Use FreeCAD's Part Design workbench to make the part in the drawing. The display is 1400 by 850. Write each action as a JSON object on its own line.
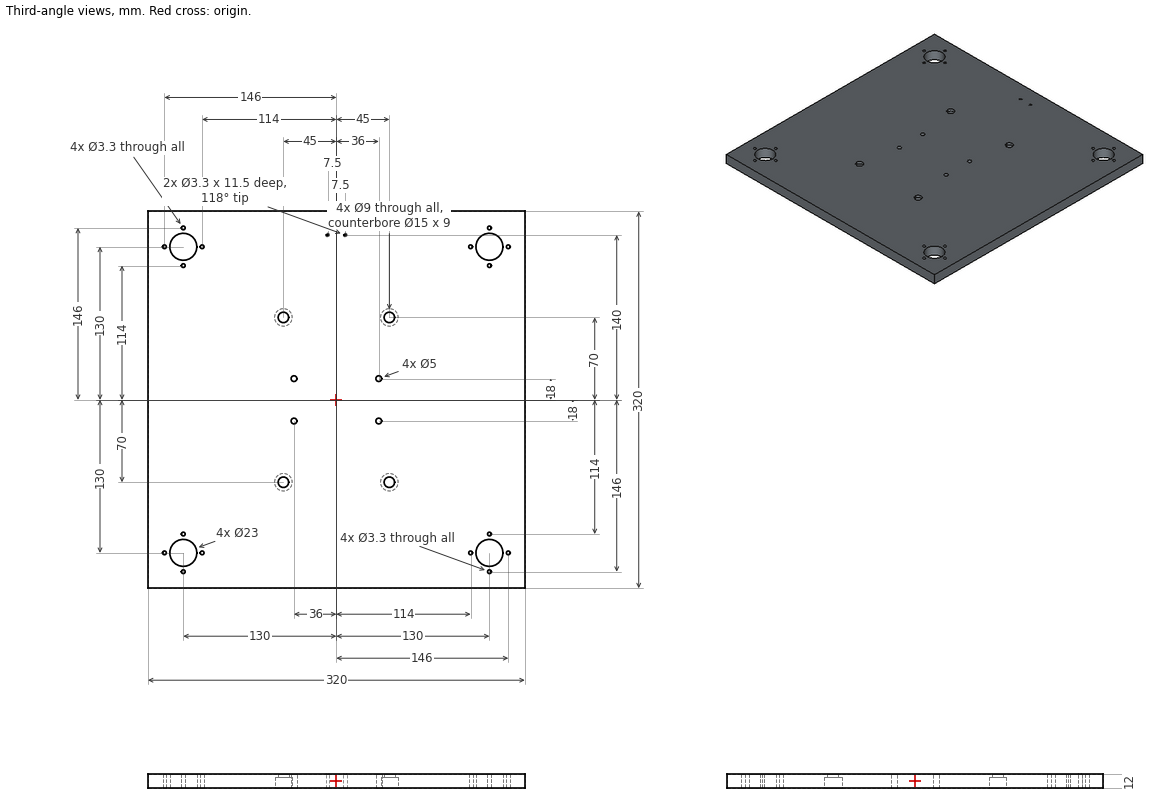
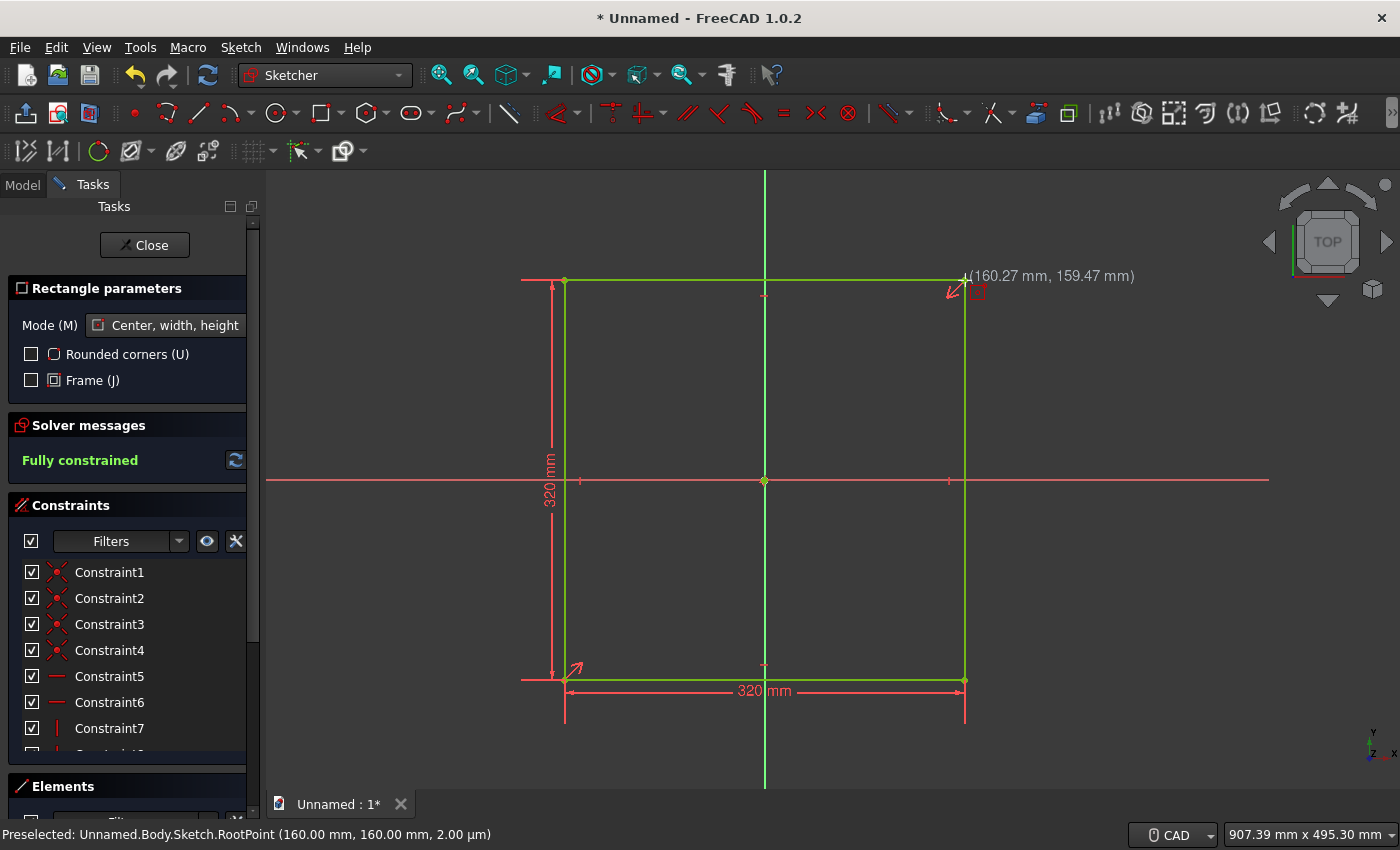
{"action": "left_click", "coordinate": [276, 114]}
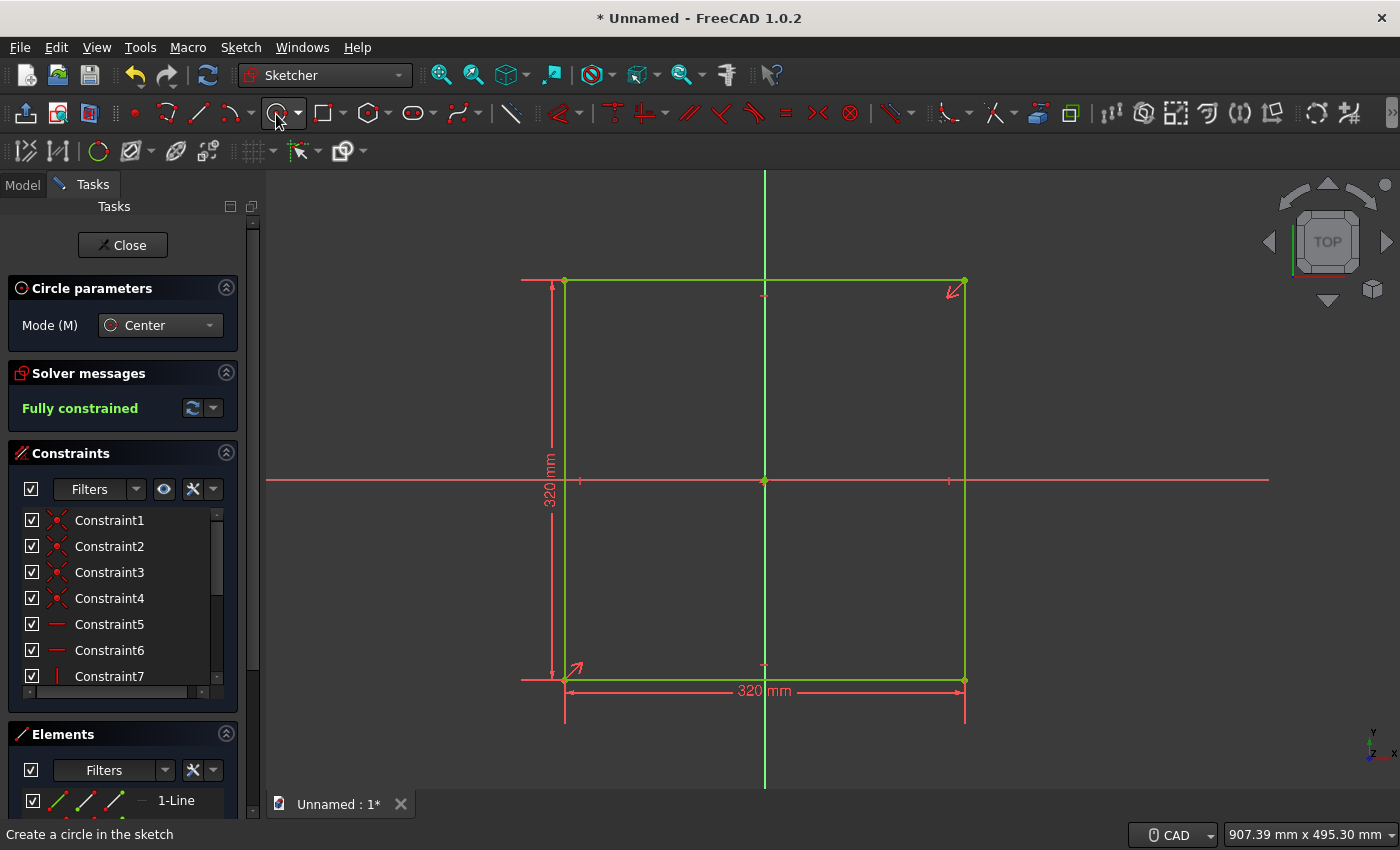
{"action": "scroll", "coordinate": [602, 643], "scroll_direction": "up", "scroll_amount": 3}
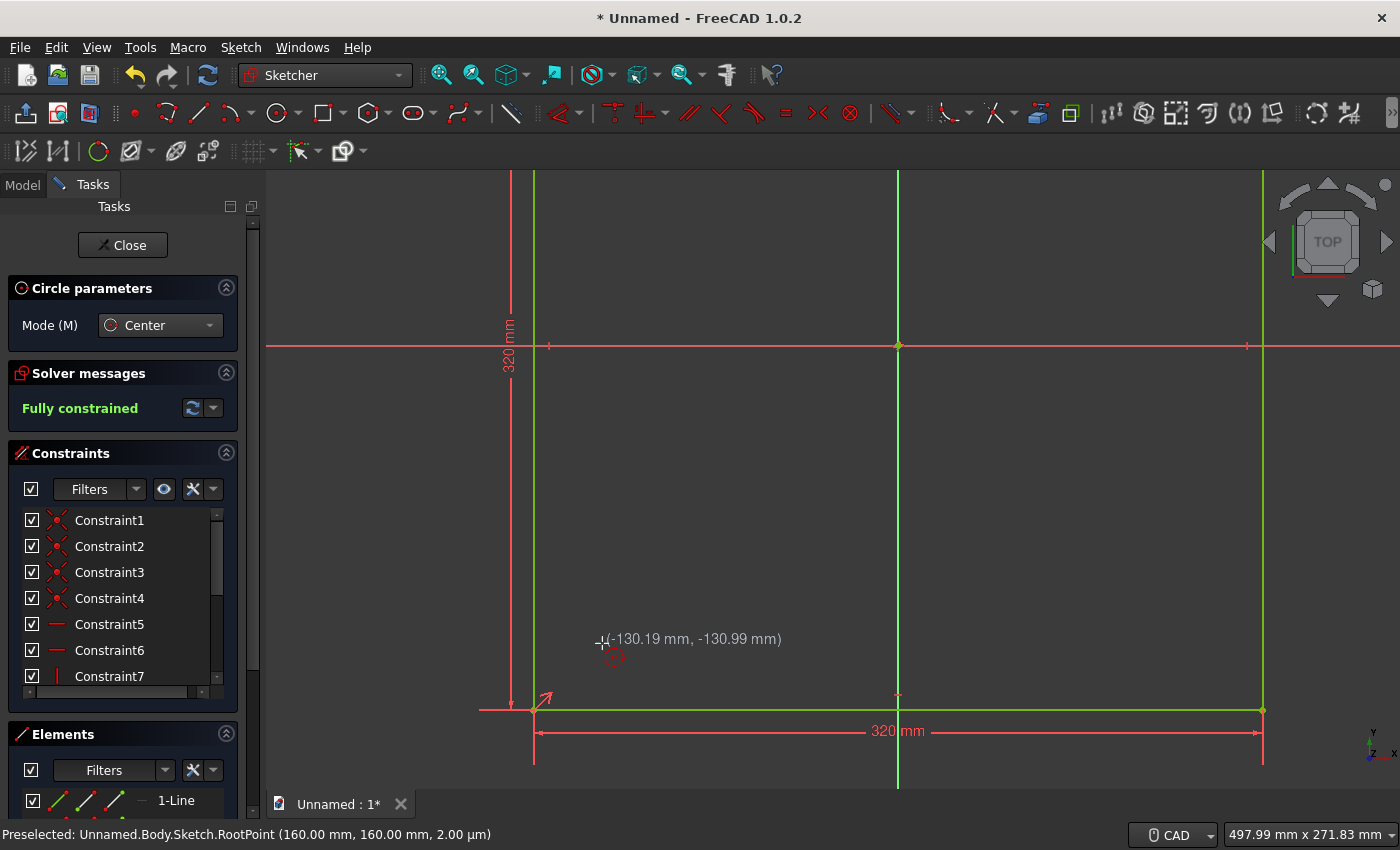
{"action": "left_click", "coordinate": [602, 642]}
{"action": "mouse_move", "coordinate": [621, 623]}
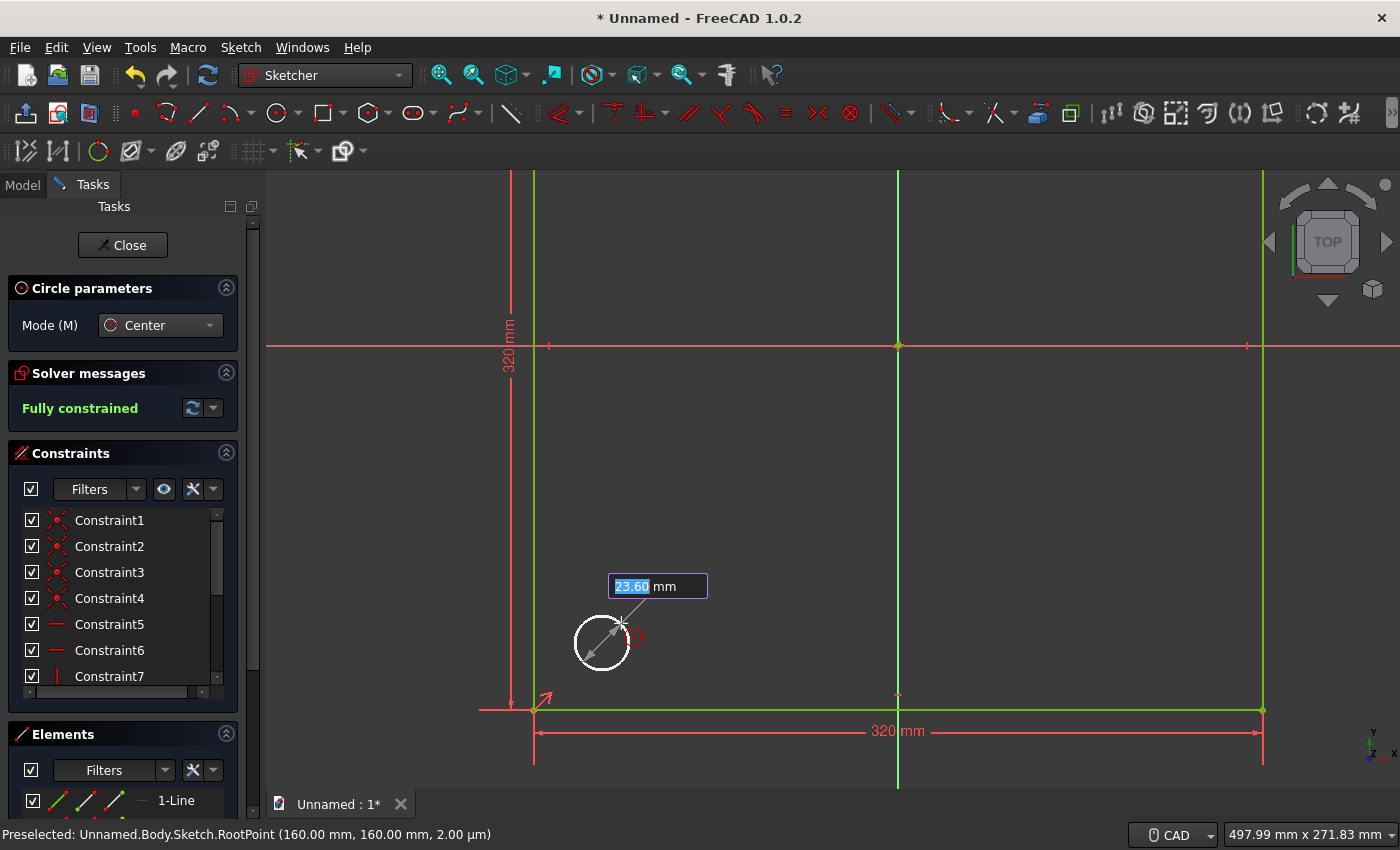
{"action": "type", "text": "23"}
{"action": "key", "text": "Return"}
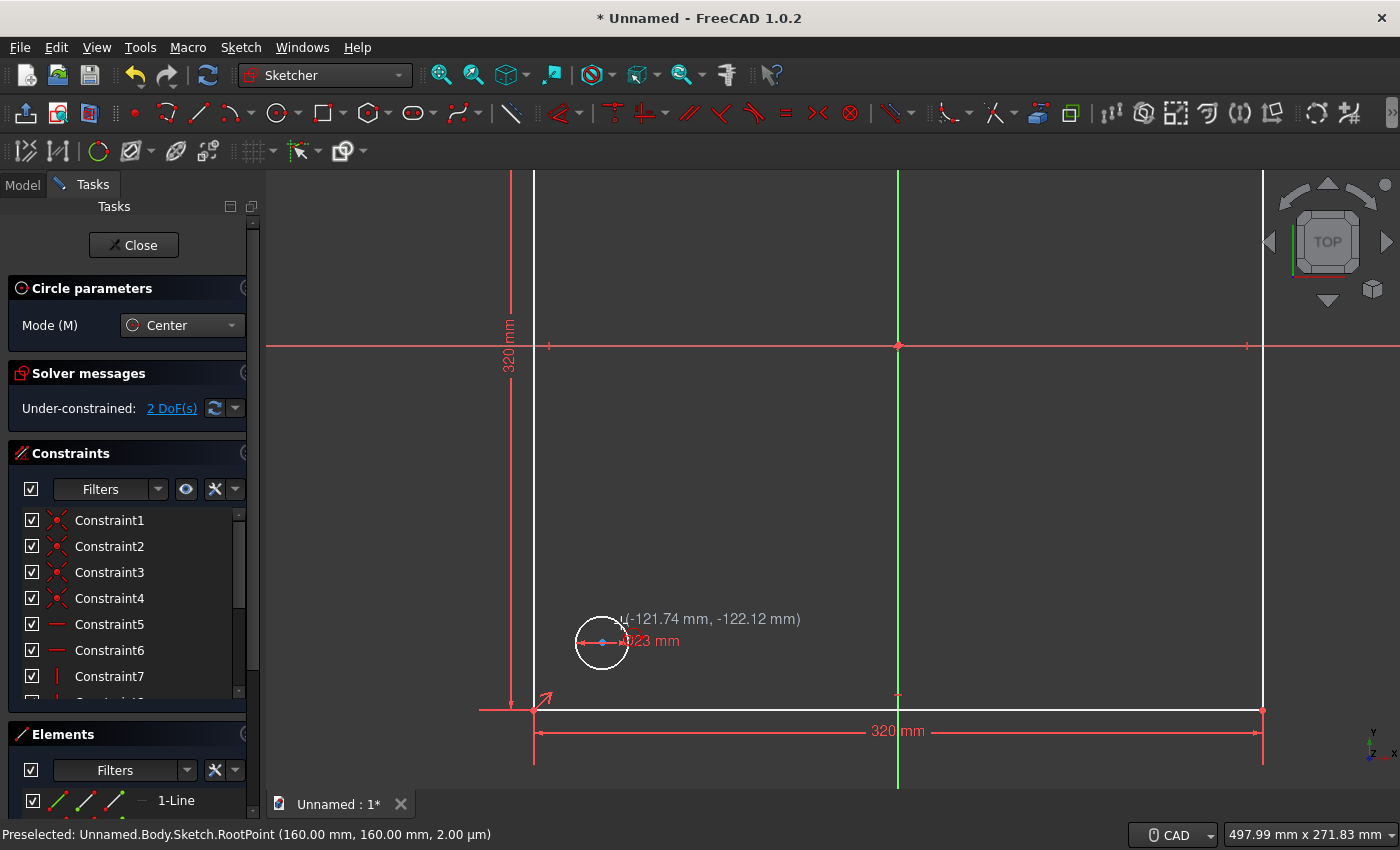
{"action": "left_click", "coordinate": [1194, 642]}
{"action": "mouse_move", "coordinate": [1213, 623]}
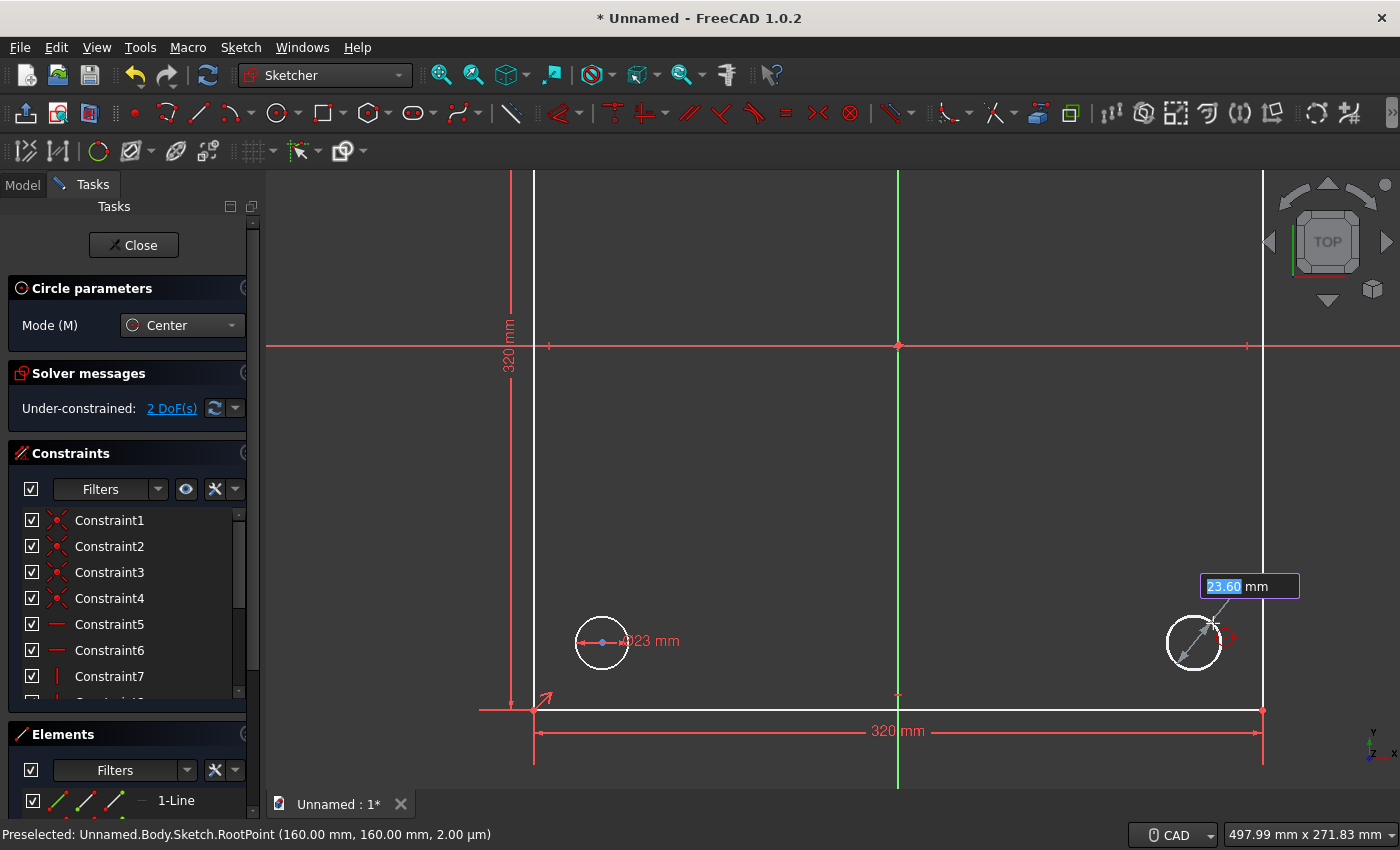
{"action": "type", "text": "23"}
{"action": "key", "text": "Return"}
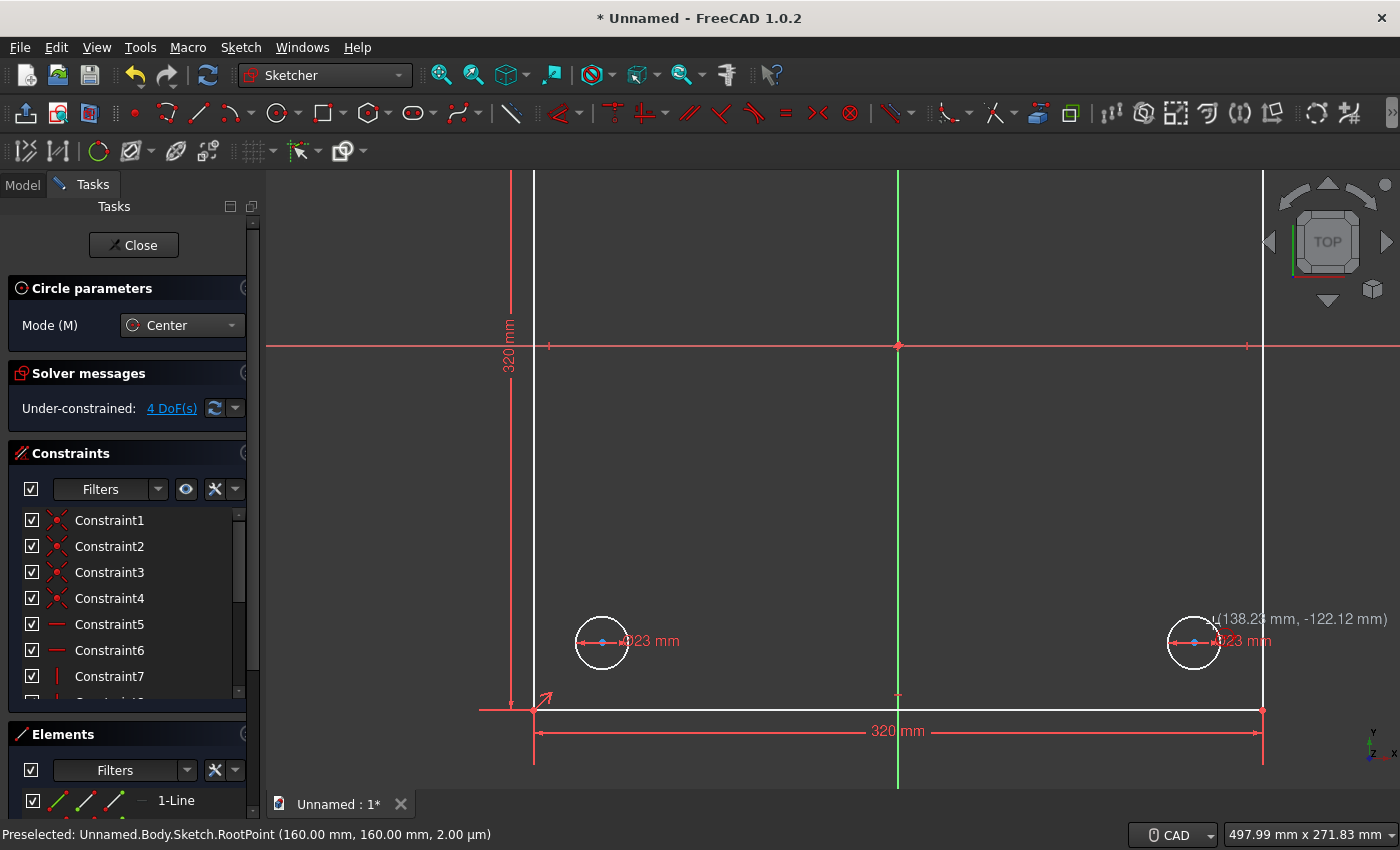
{"action": "scroll", "coordinate": [602, 642], "scroll_direction": "down", "scroll_amount": 3}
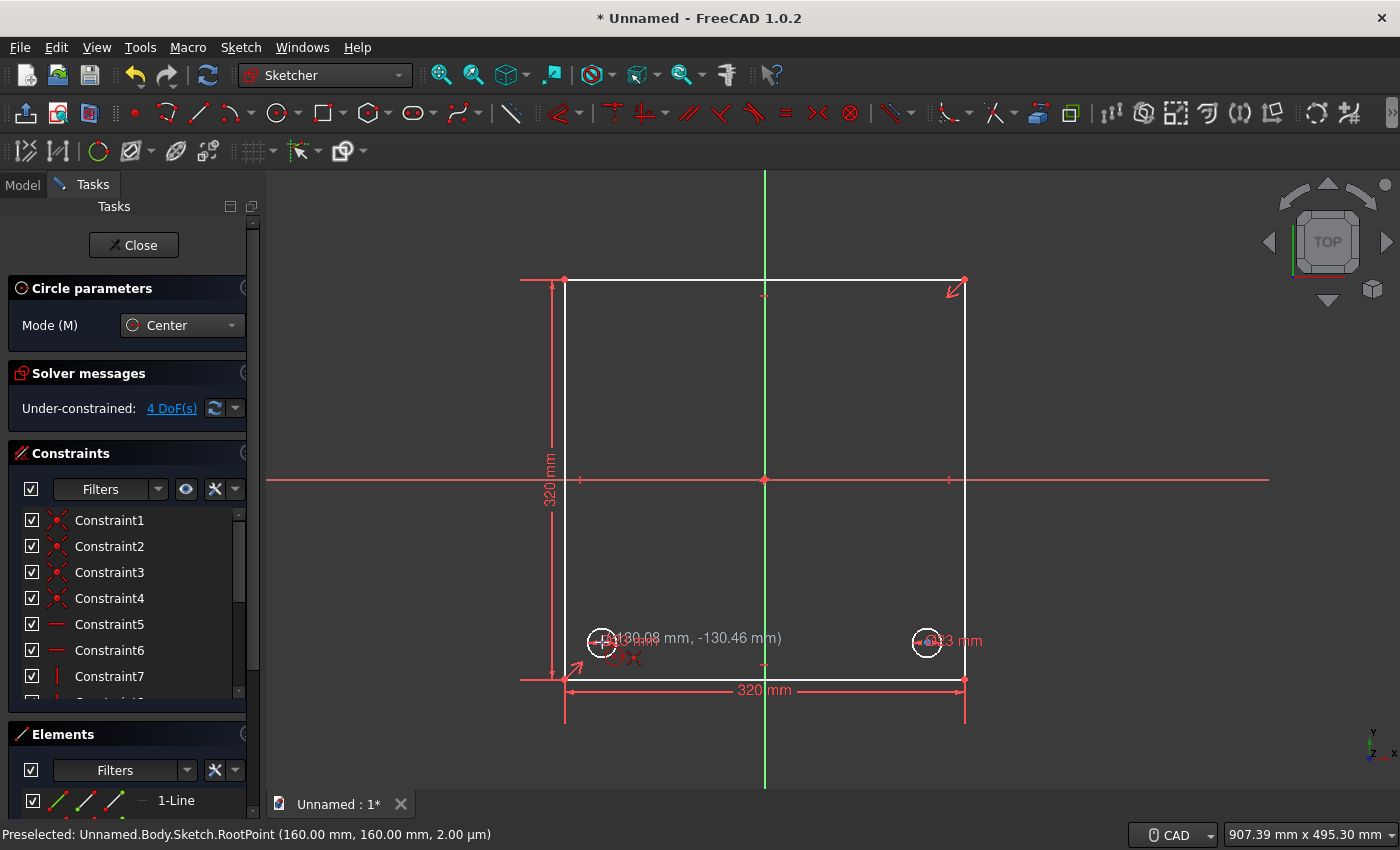
{"action": "scroll", "coordinate": [602, 317], "scroll_direction": "up", "scroll_amount": 3}